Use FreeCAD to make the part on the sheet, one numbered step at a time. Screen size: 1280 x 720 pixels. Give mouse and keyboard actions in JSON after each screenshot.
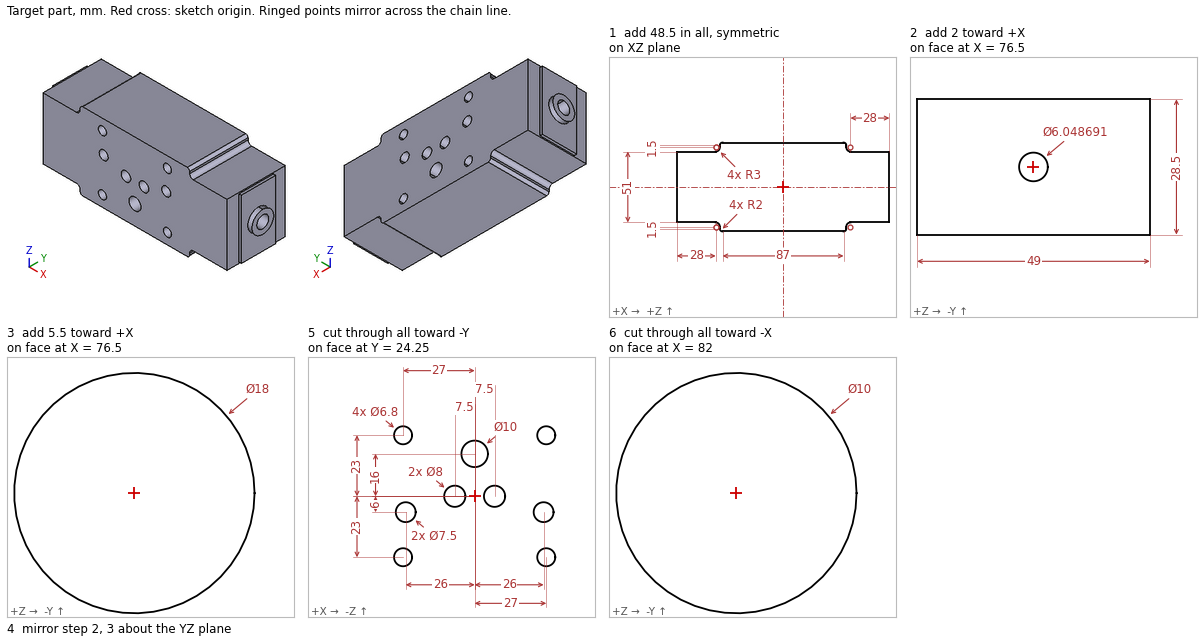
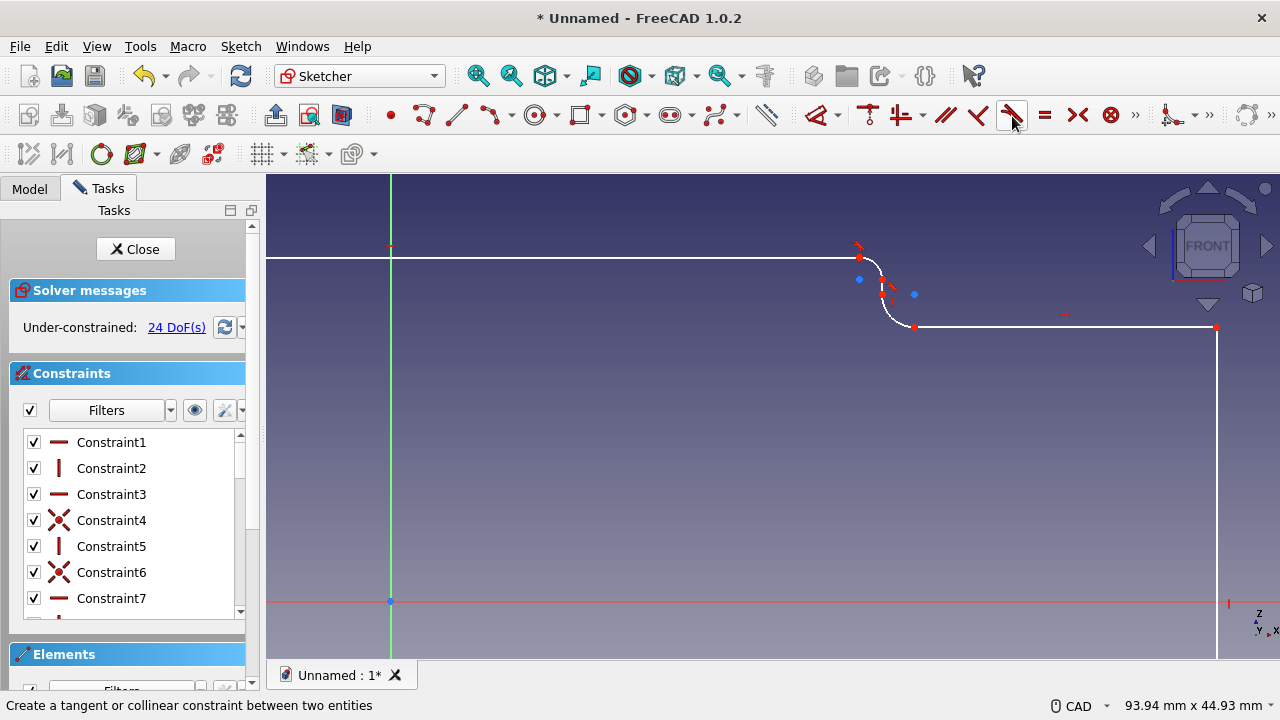
{"action": "left_click", "coordinate": [1005, 327]}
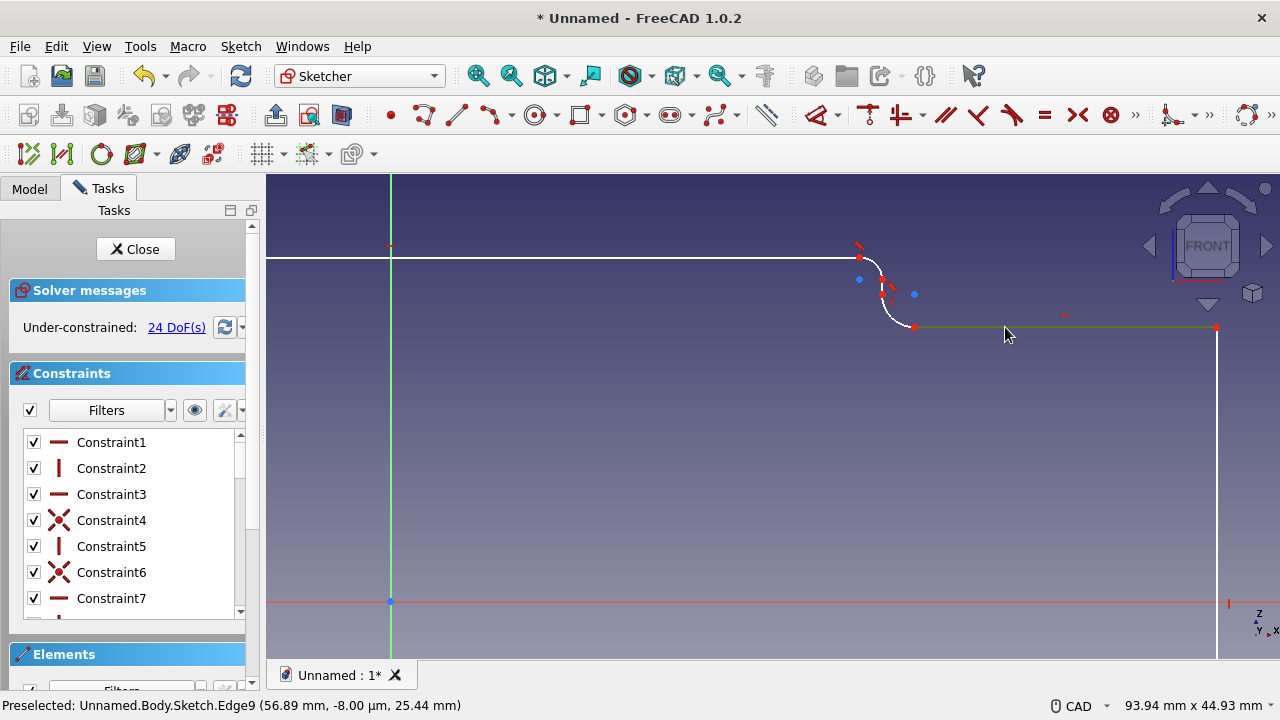
{"action": "left_click", "coordinate": [886, 310]}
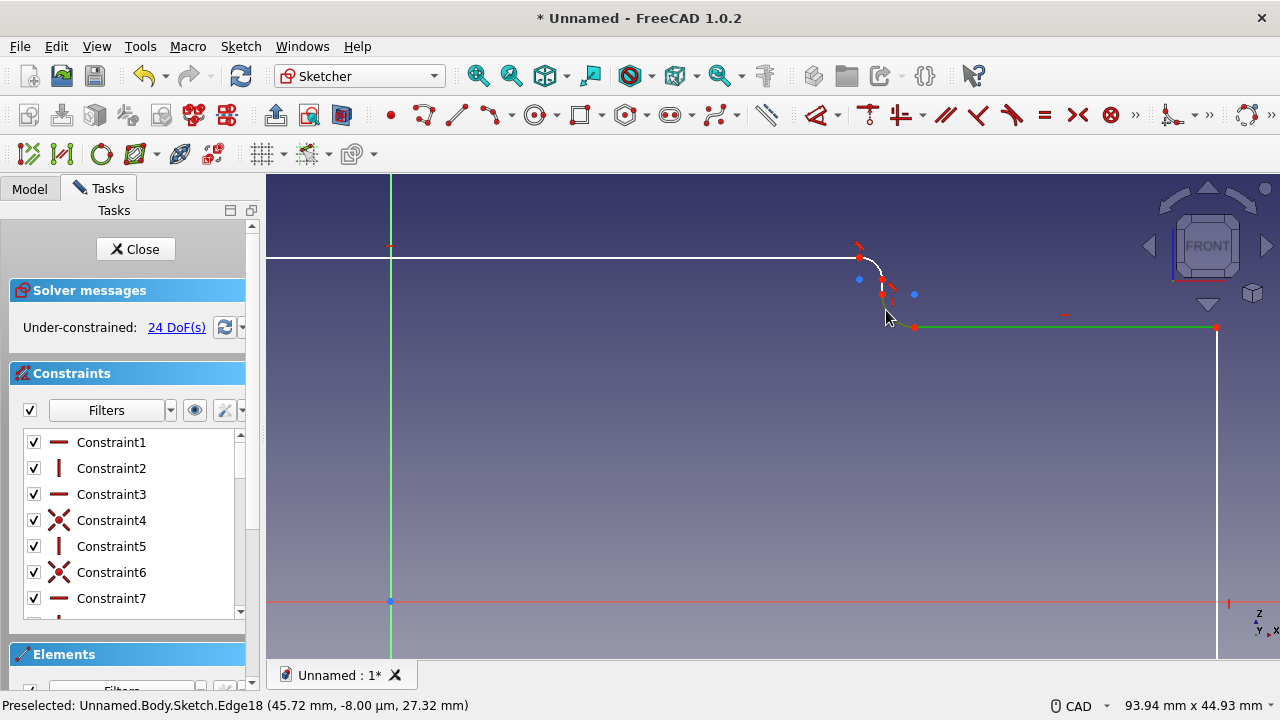
{"action": "left_click", "coordinate": [1012, 116]}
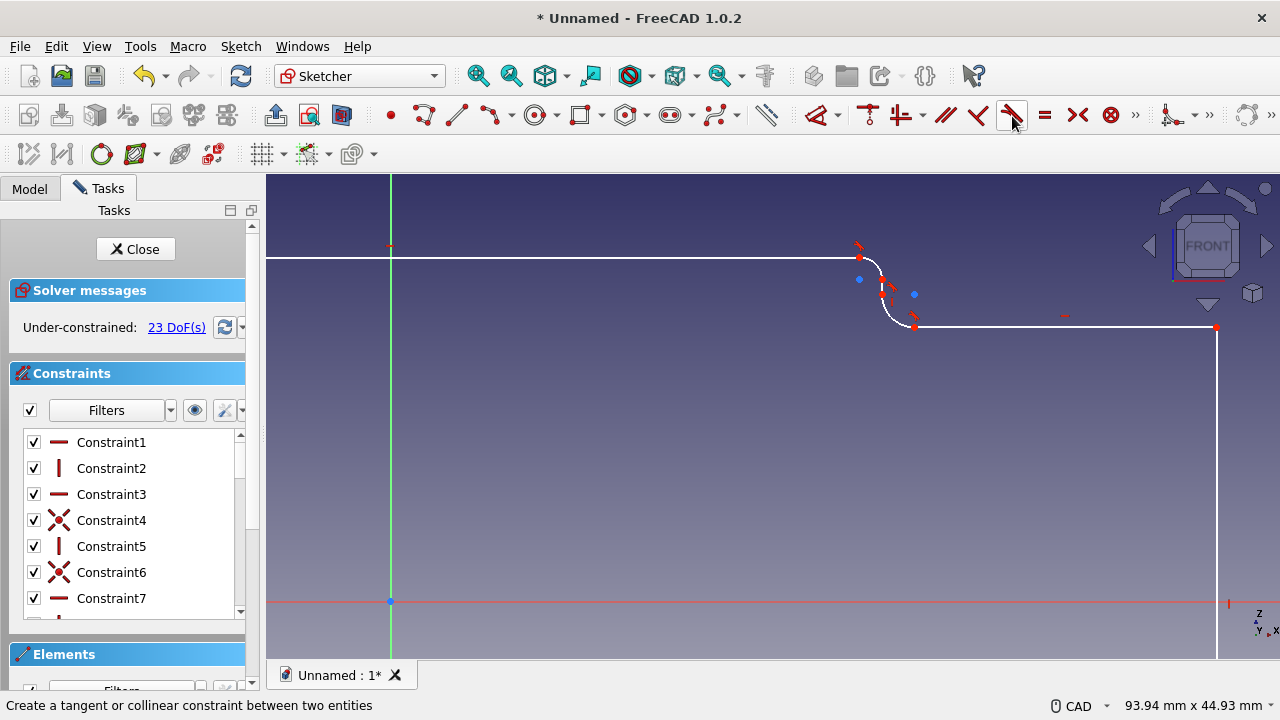
{"action": "scroll", "coordinate": [887, 309], "scroll_direction": "down", "scroll_amount": 5}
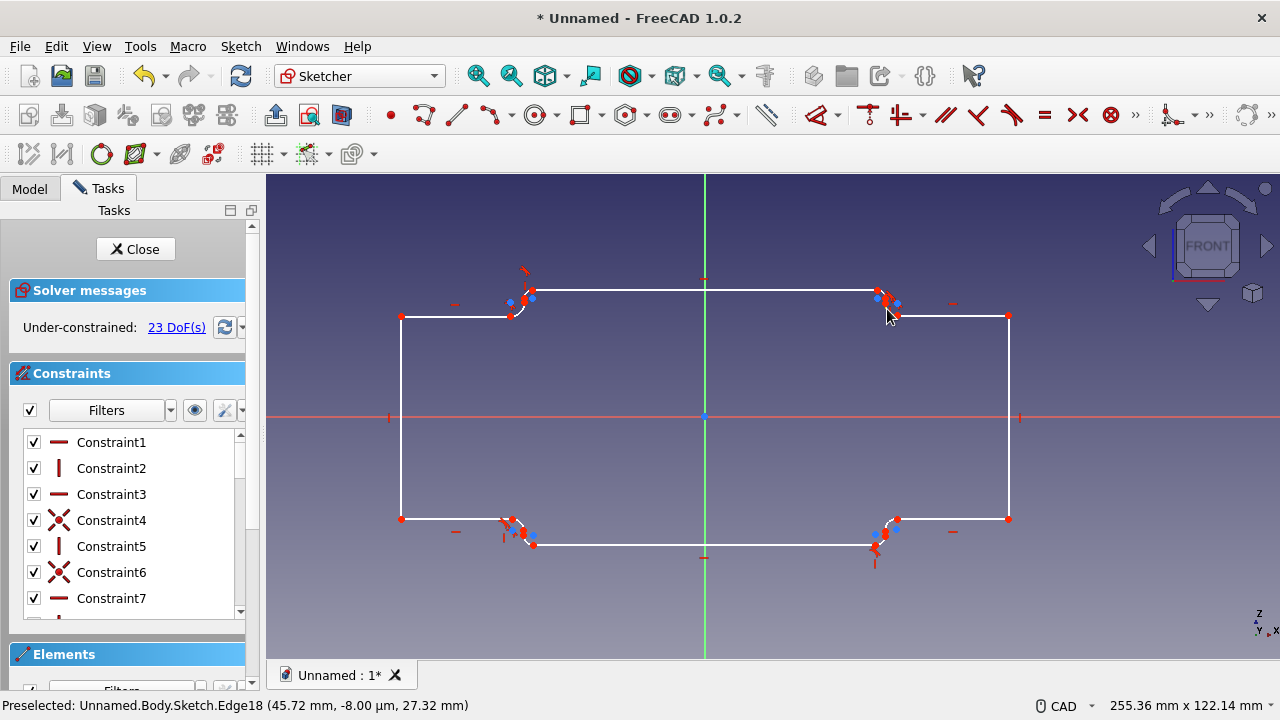
{"action": "left_click", "coordinate": [975, 519]}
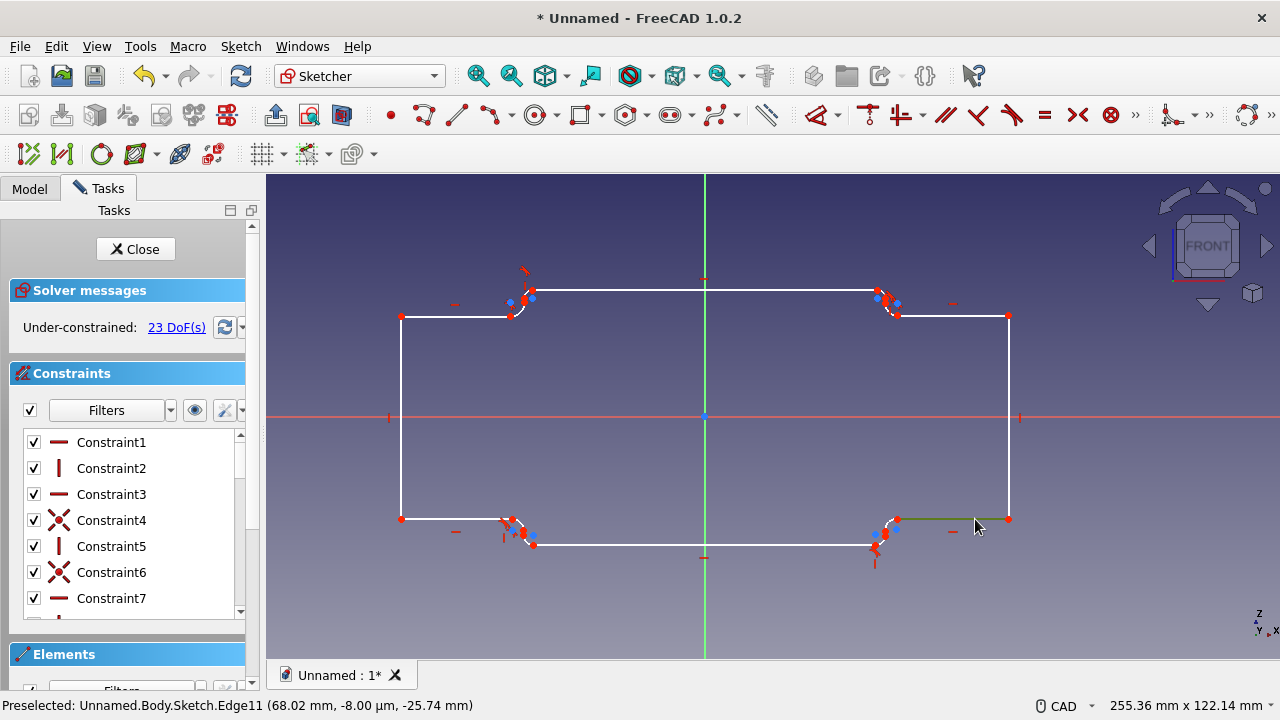
{"action": "scroll", "coordinate": [889, 522], "scroll_direction": "up", "scroll_amount": 2}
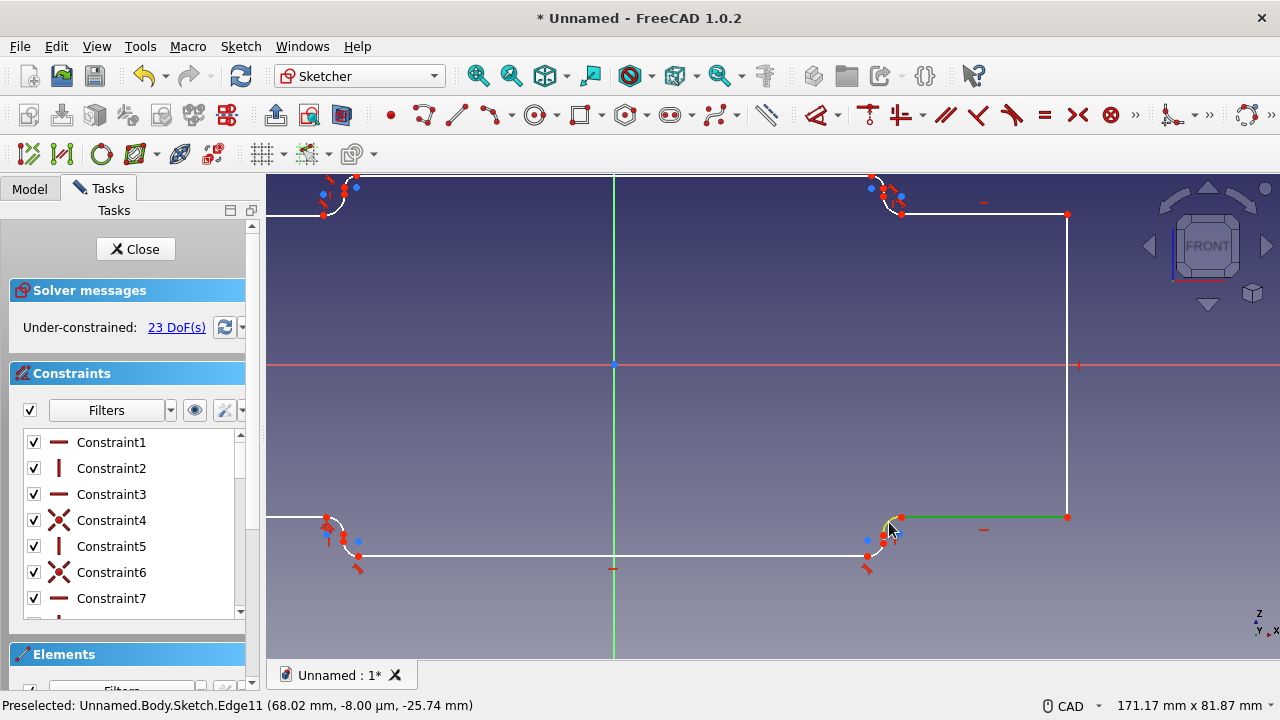
{"action": "left_click", "coordinate": [888, 522]}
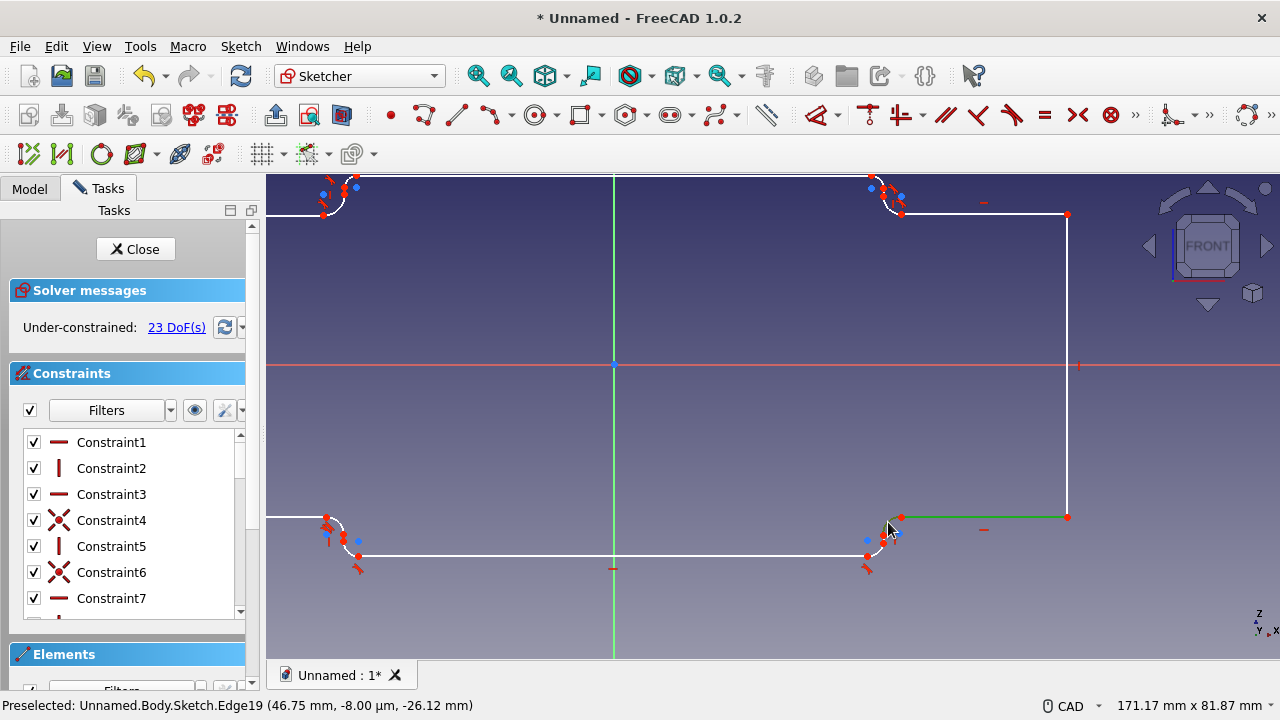
{"action": "left_click", "coordinate": [1012, 116]}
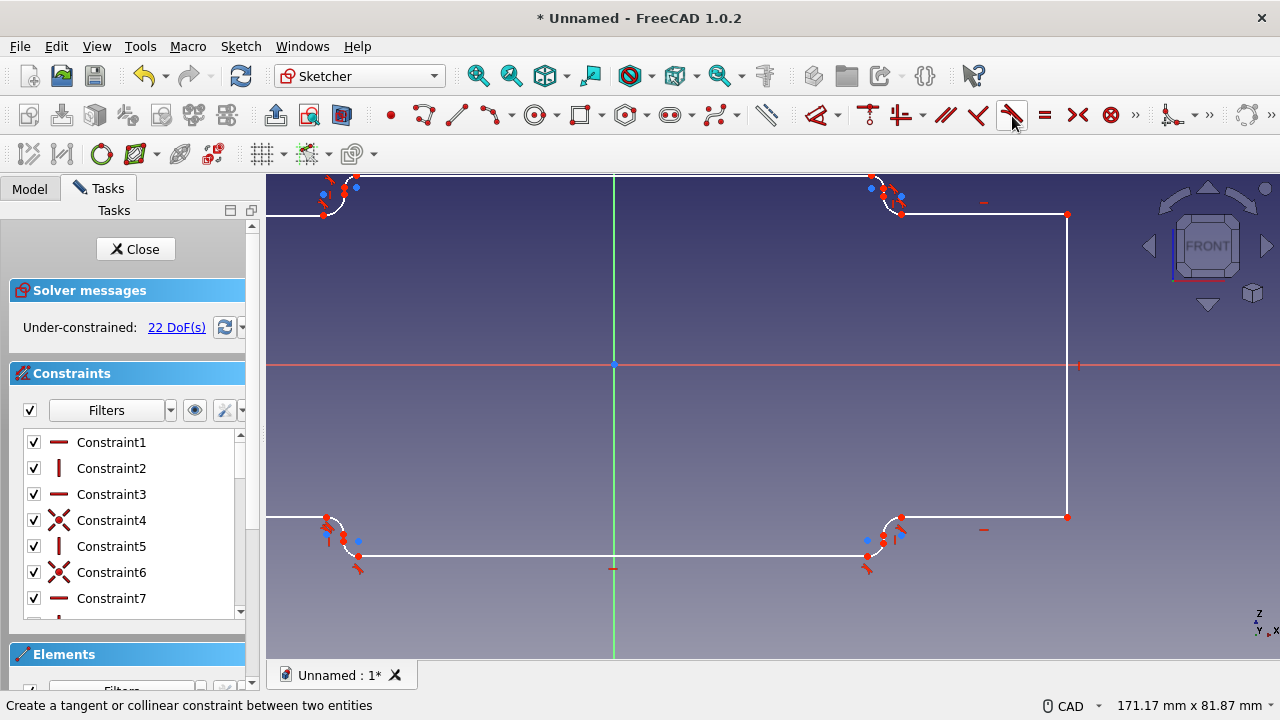
{"action": "scroll", "coordinate": [884, 539], "scroll_direction": "up", "scroll_amount": 7}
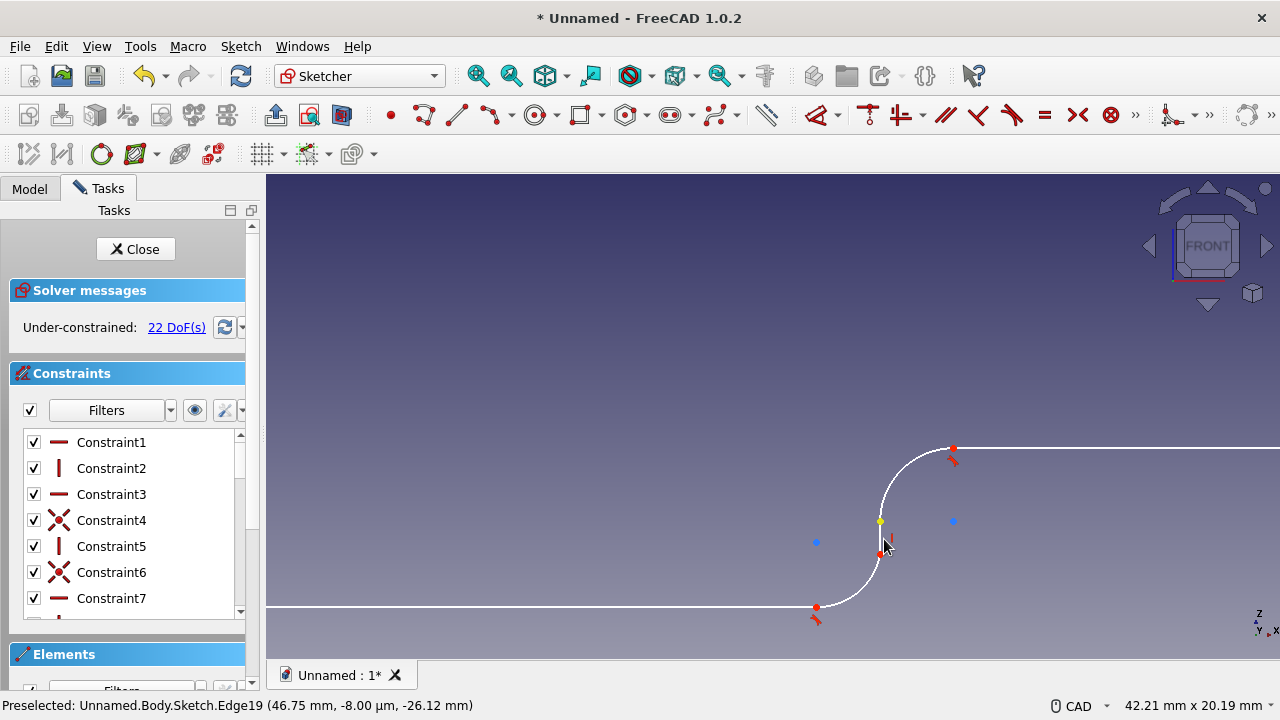
{"action": "left_click", "coordinate": [880, 538]}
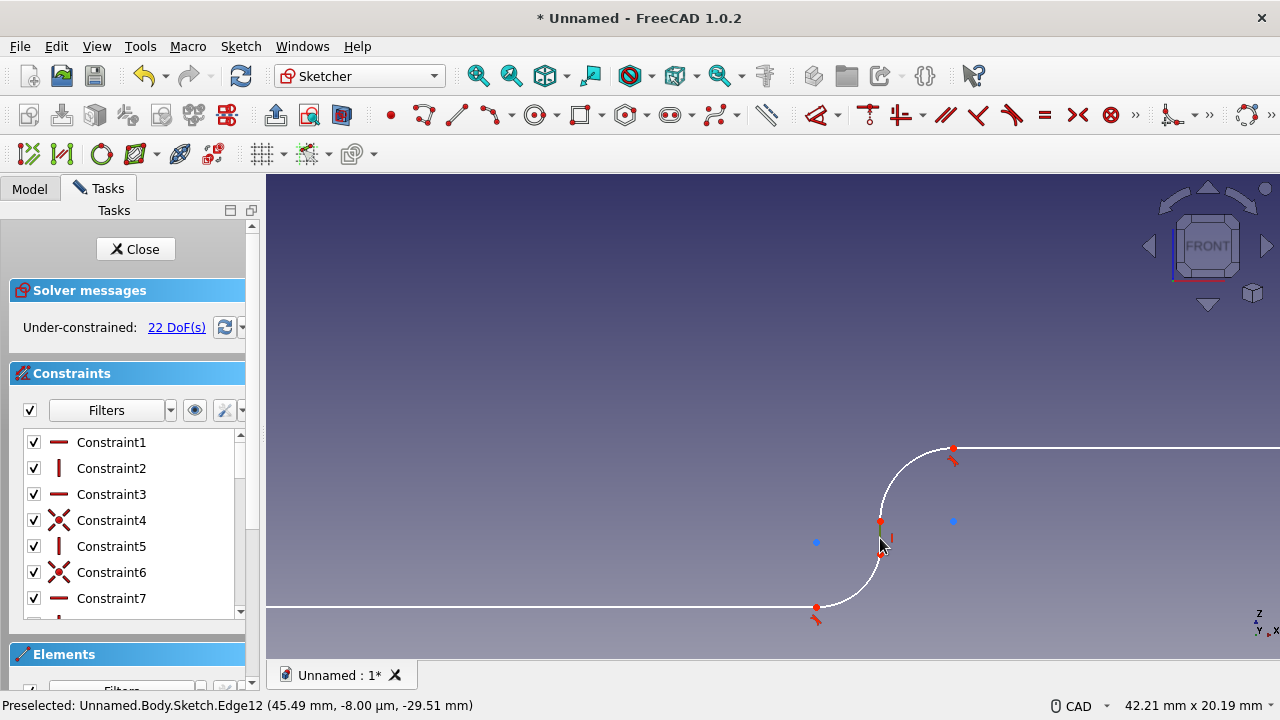
{"action": "left_click", "coordinate": [921, 456]}